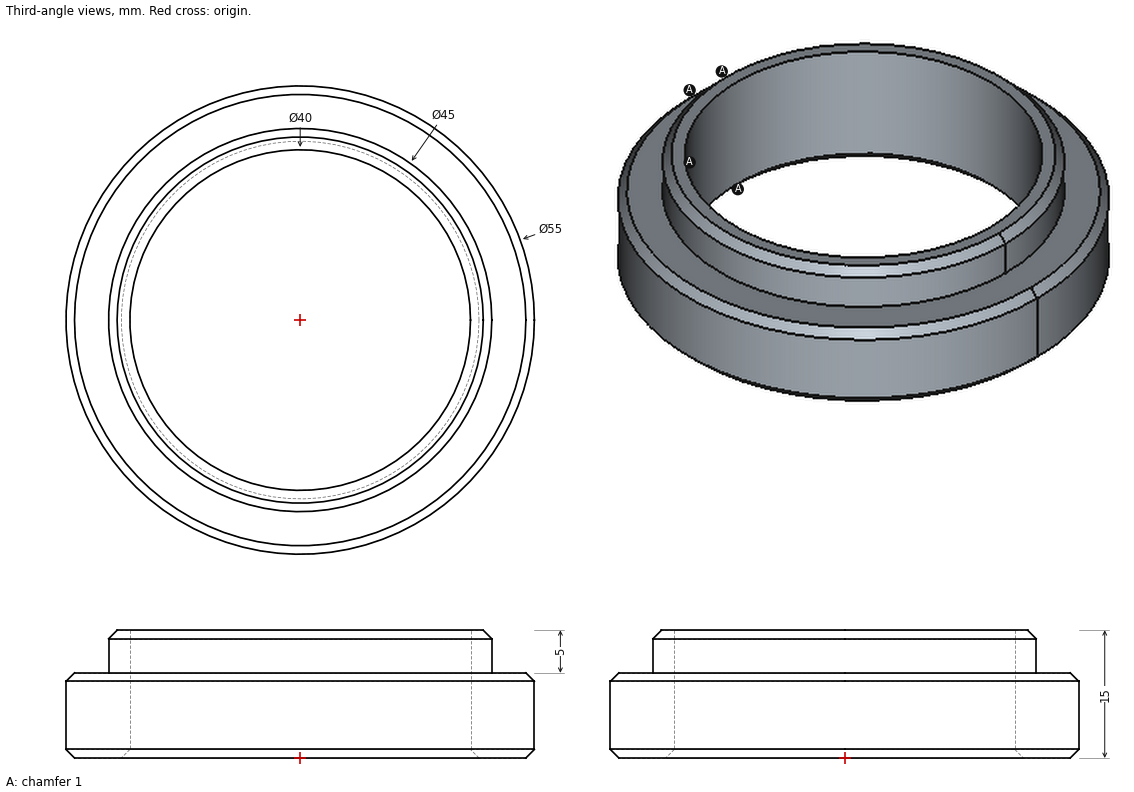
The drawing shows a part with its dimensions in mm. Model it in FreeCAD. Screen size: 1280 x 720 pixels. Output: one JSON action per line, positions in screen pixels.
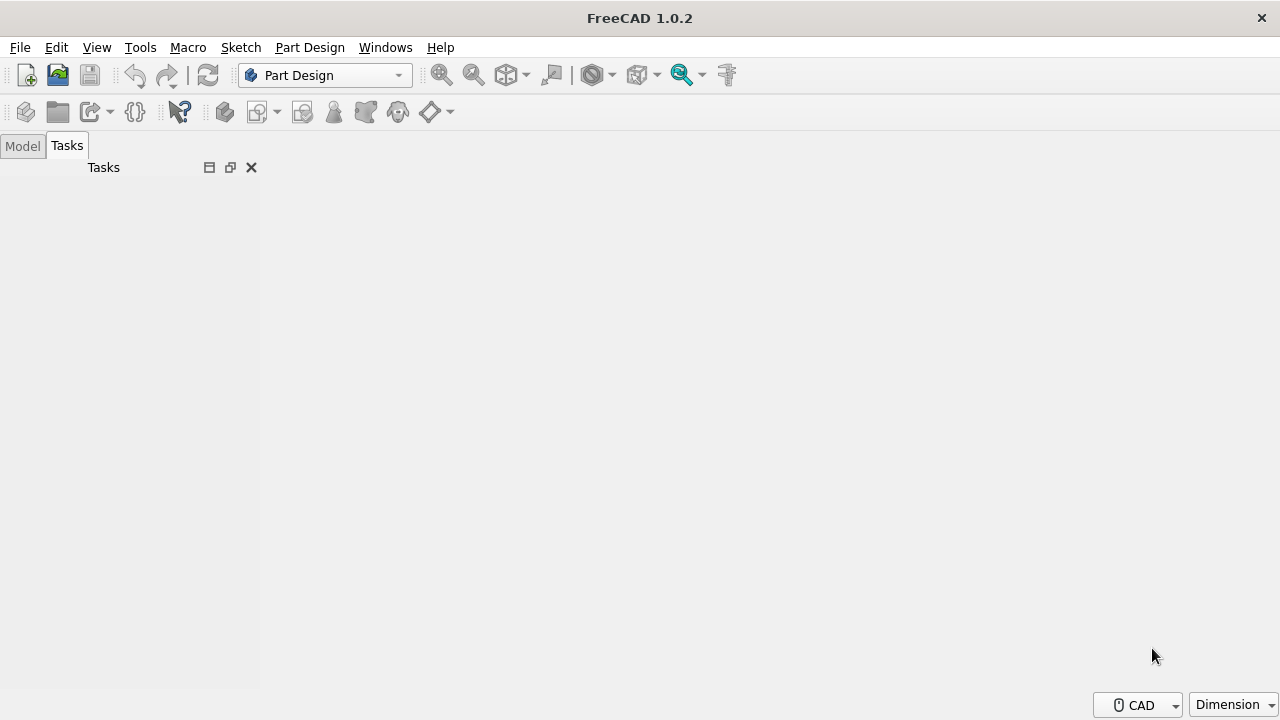
{"action": "key", "text": "ctrl+n"}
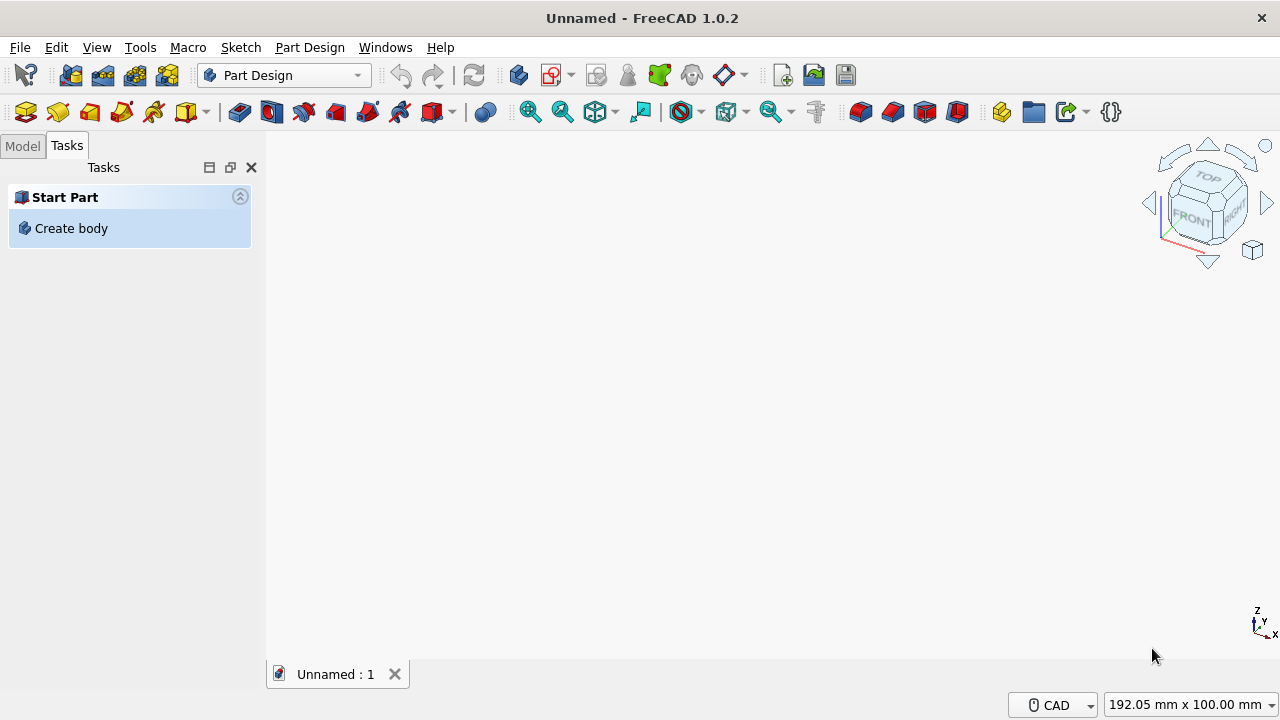
{"action": "left_click", "coordinate": [552, 76]}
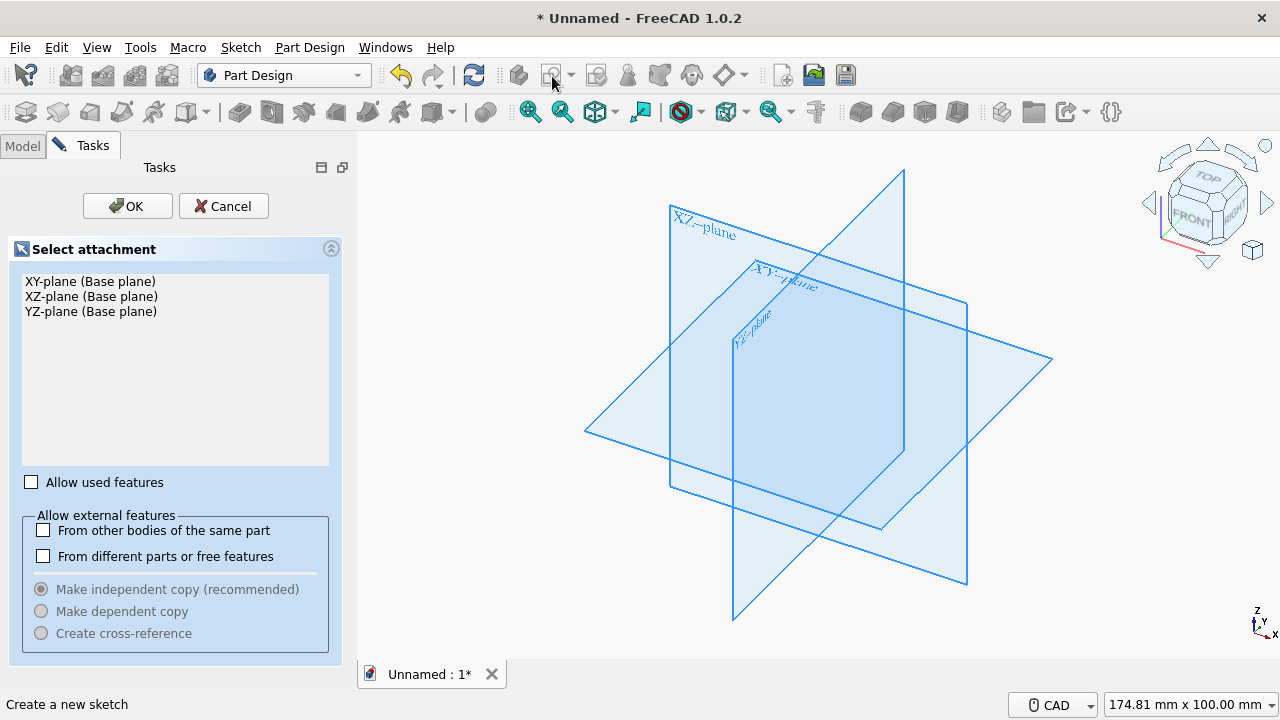
{"action": "left_click", "coordinate": [82, 282]}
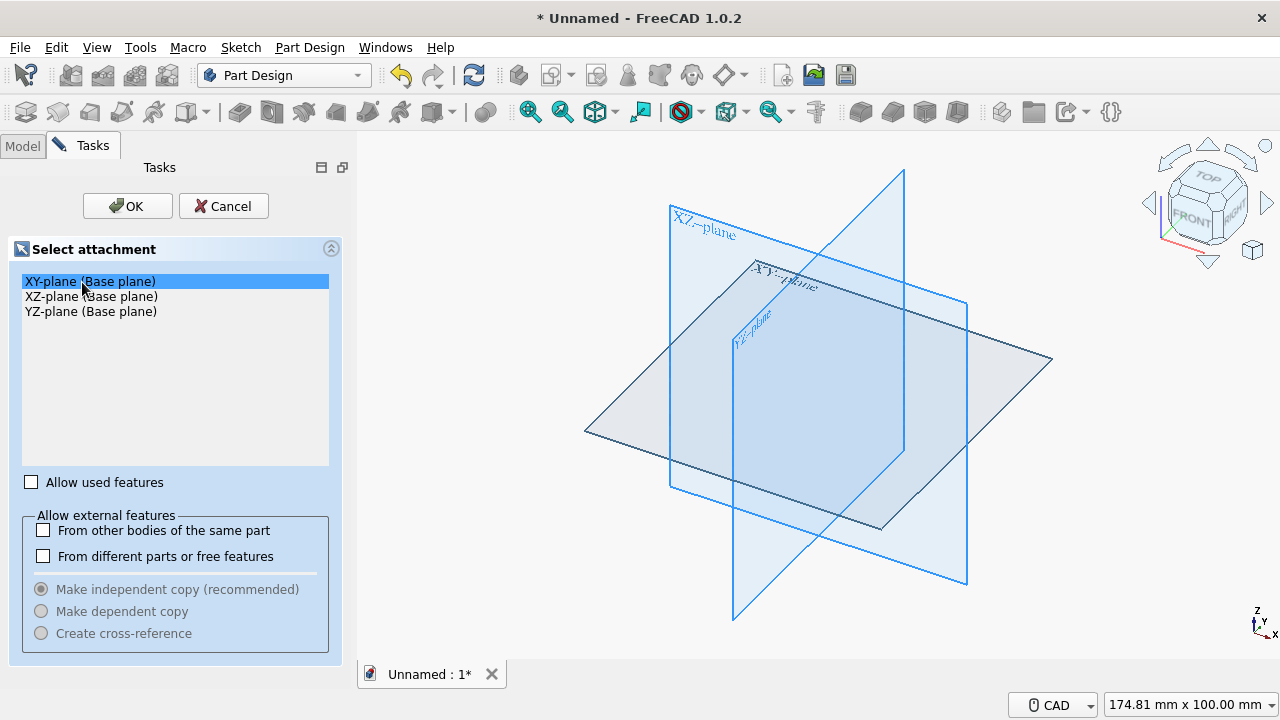
{"action": "left_click", "coordinate": [128, 206]}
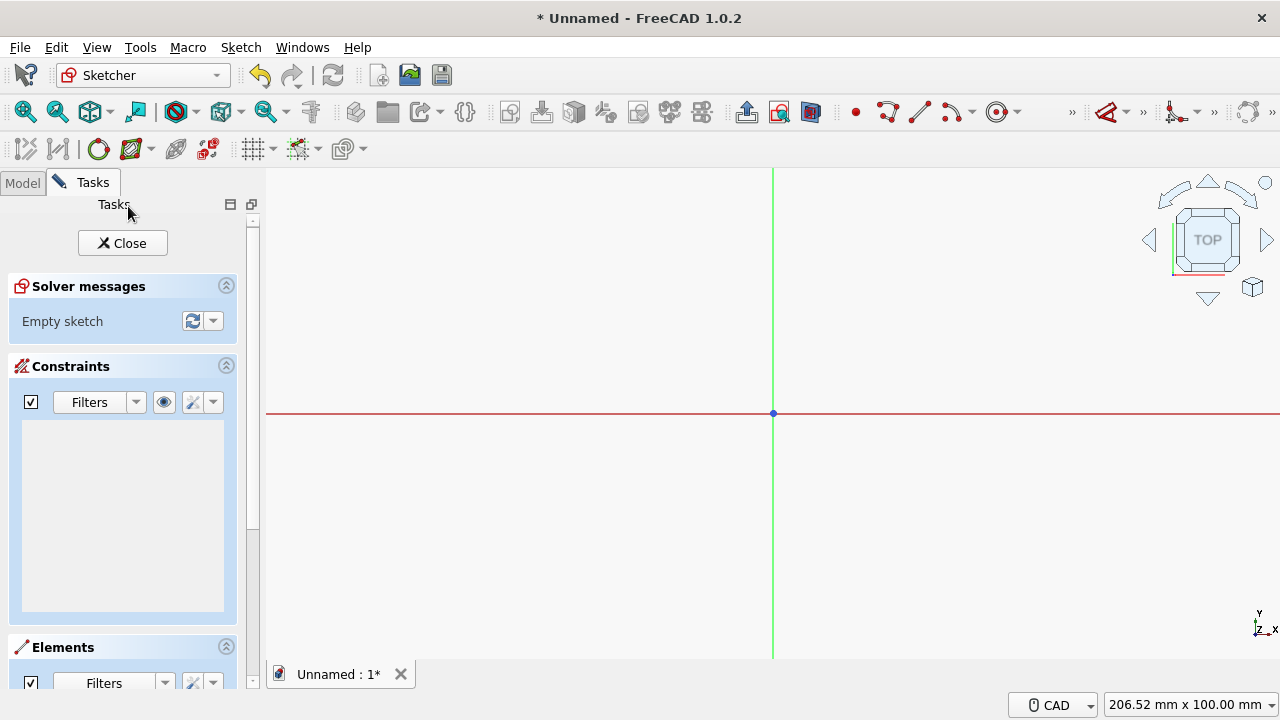
{"action": "key", "text": "g c"}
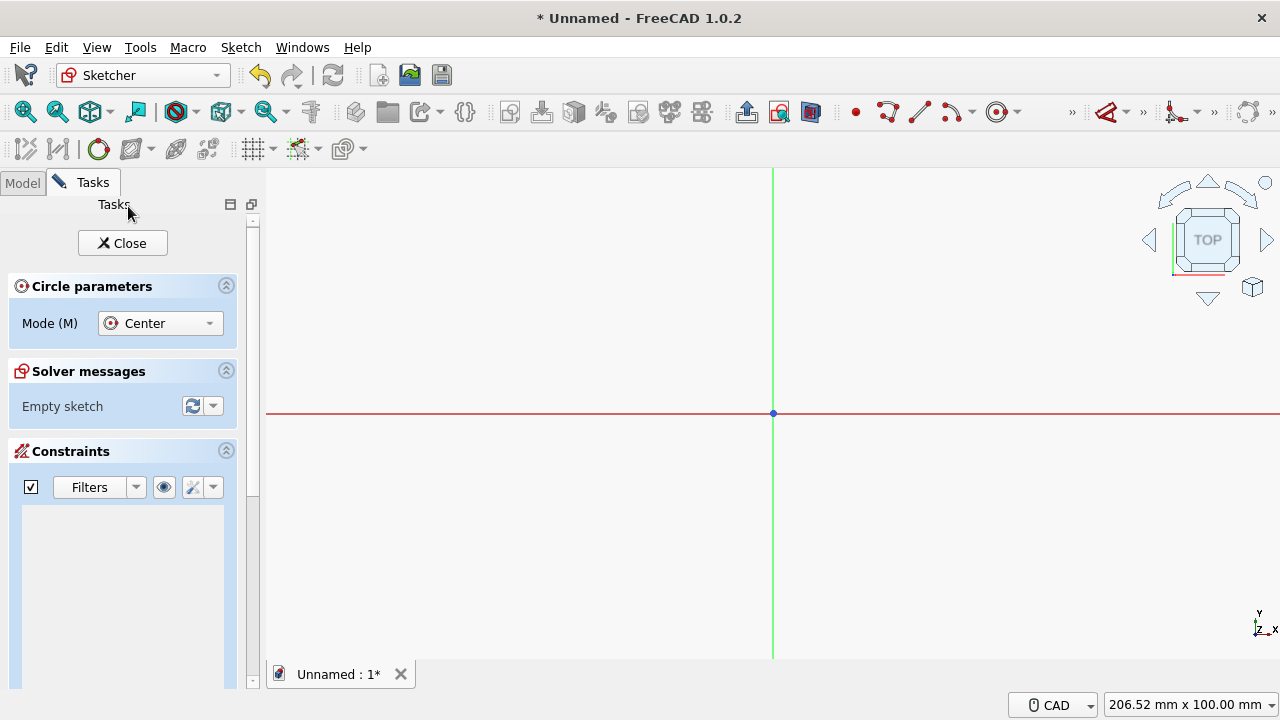
{"action": "left_click", "coordinate": [773, 414]}
{"action": "mouse_move", "coordinate": [868, 318]}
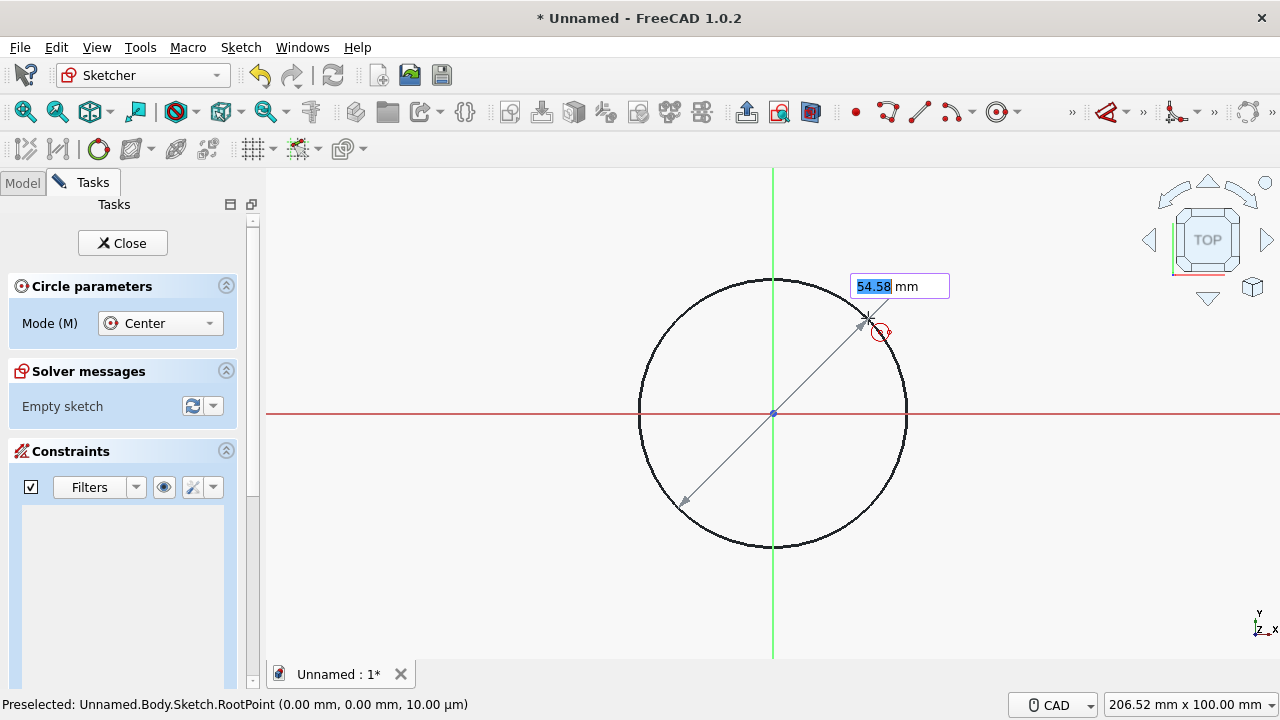
{"action": "type", "text": "55"}
{"action": "key", "text": "Return"}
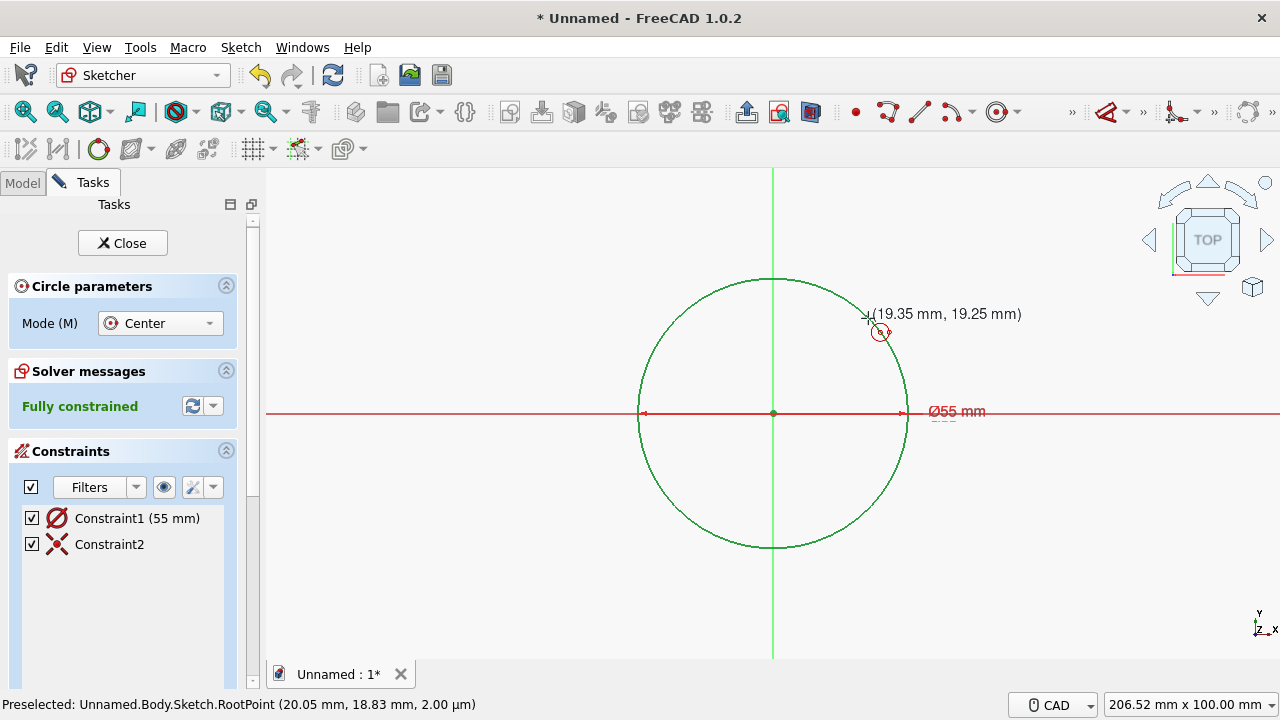
{"action": "left_click", "coordinate": [773, 414]}
{"action": "mouse_move", "coordinate": [842, 344]}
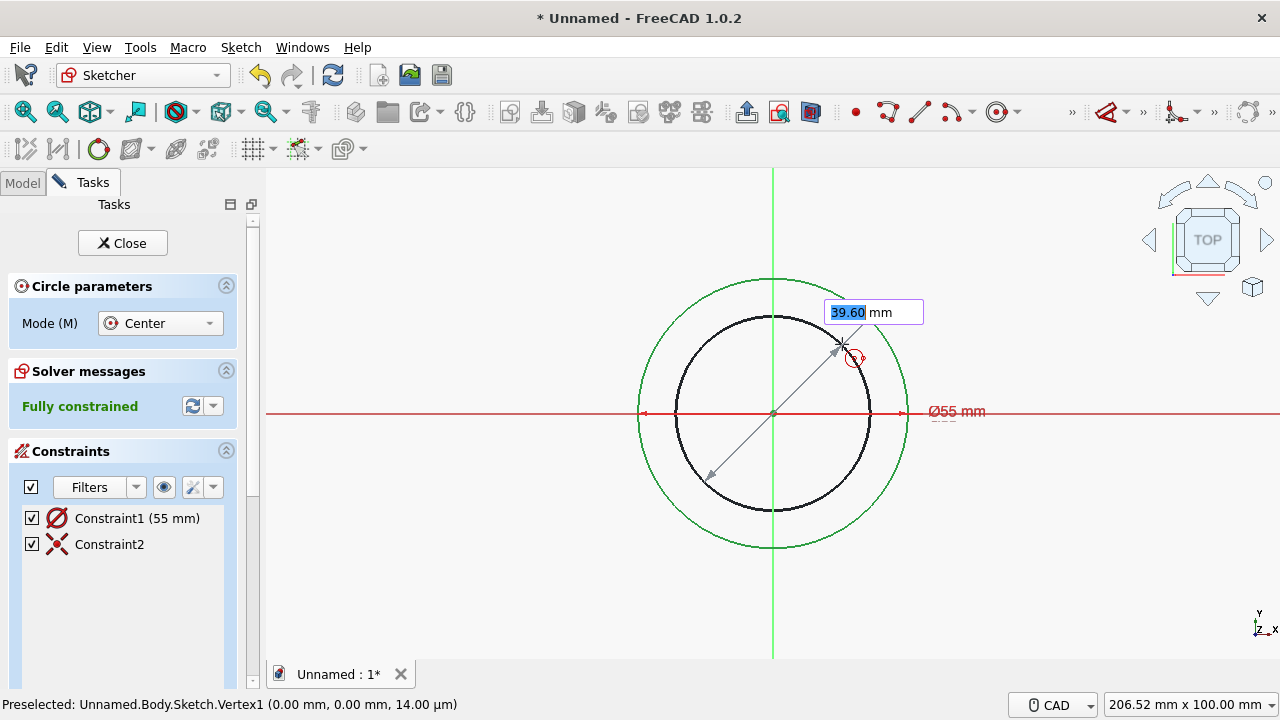
{"action": "type", "text": "40"}
{"action": "key", "text": "Return"}
{"action": "key", "text": "Escape"}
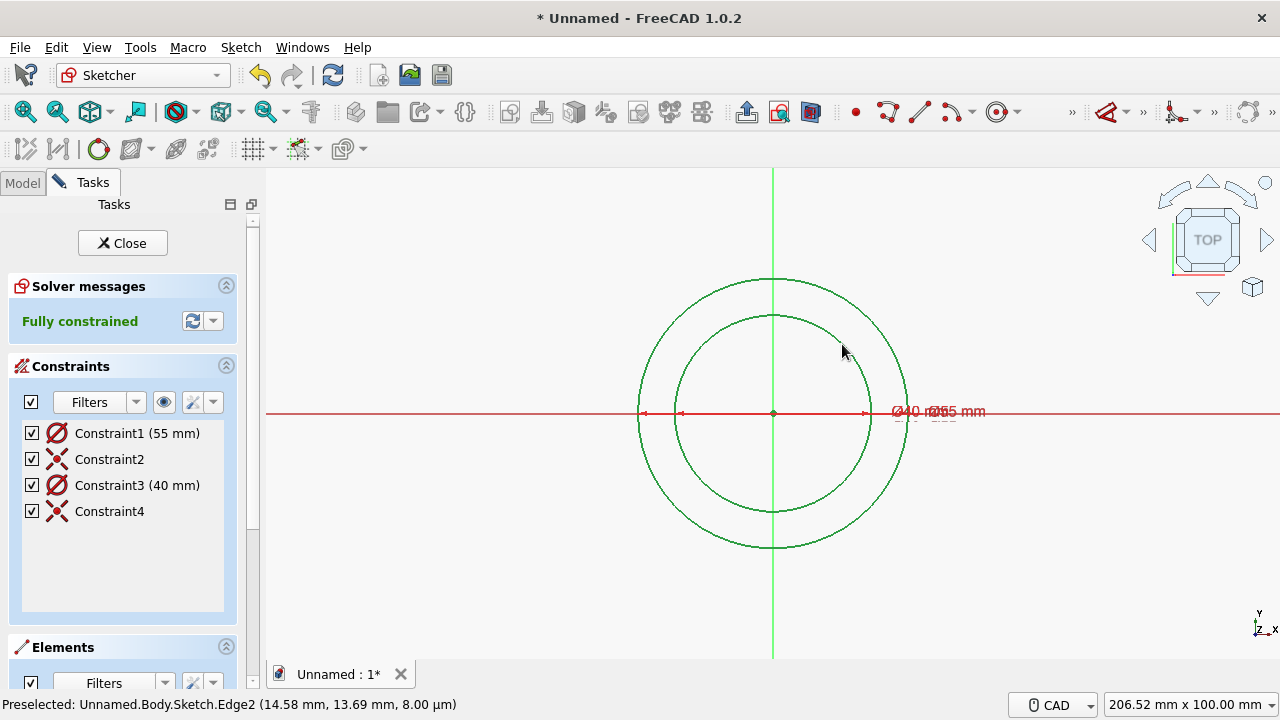
{"action": "left_click", "coordinate": [123, 243]}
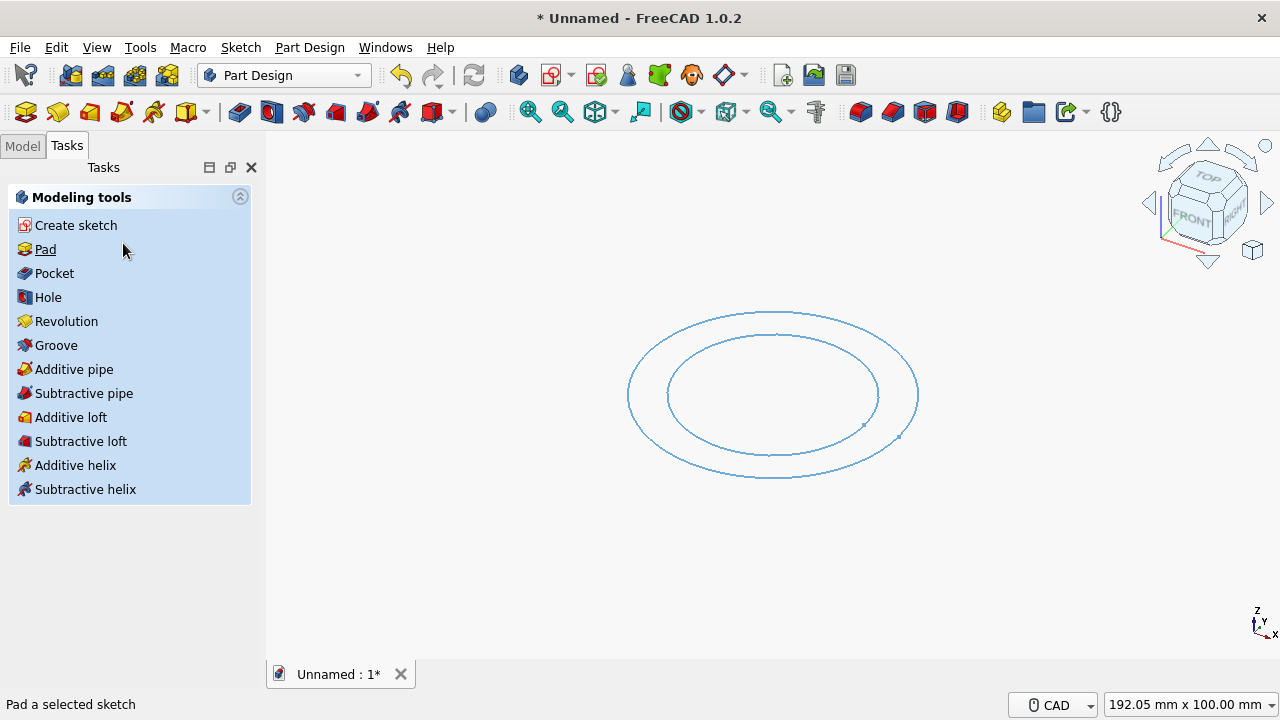
{"action": "left_click", "coordinate": [26, 112]}